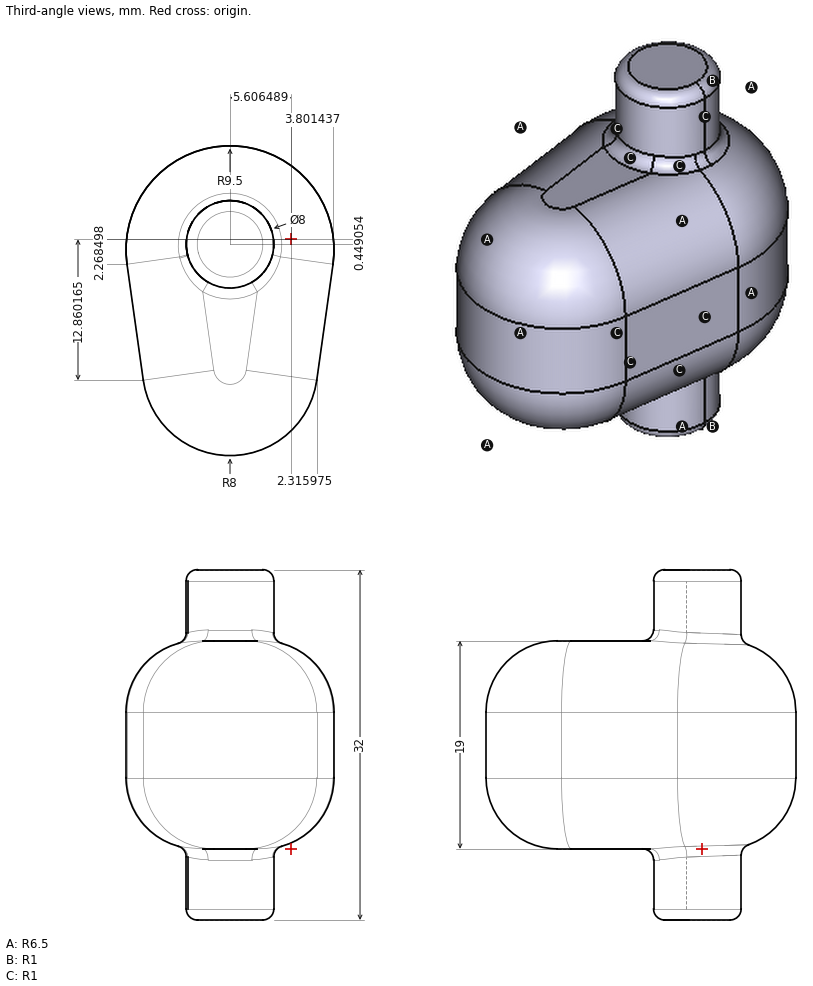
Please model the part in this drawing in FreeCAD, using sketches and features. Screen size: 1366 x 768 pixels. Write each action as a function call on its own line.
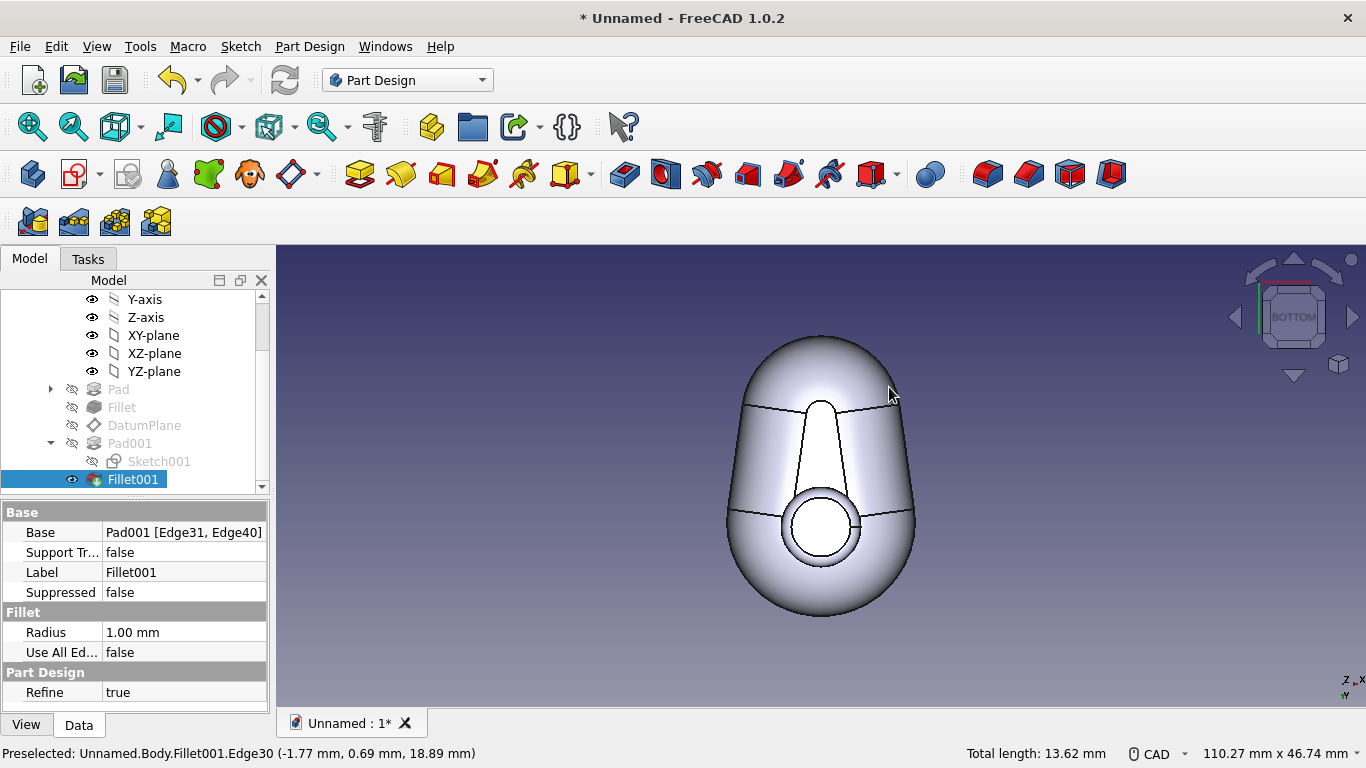
key(4)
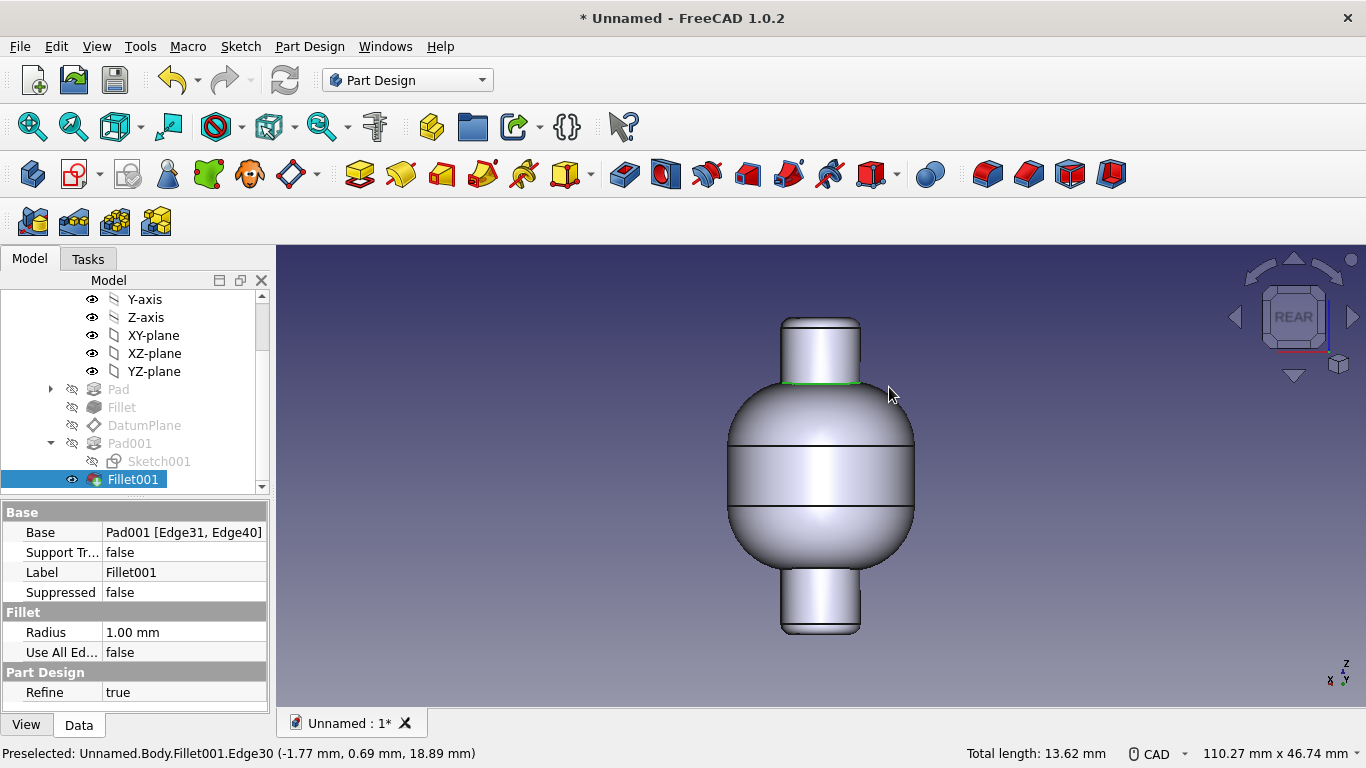
key(6)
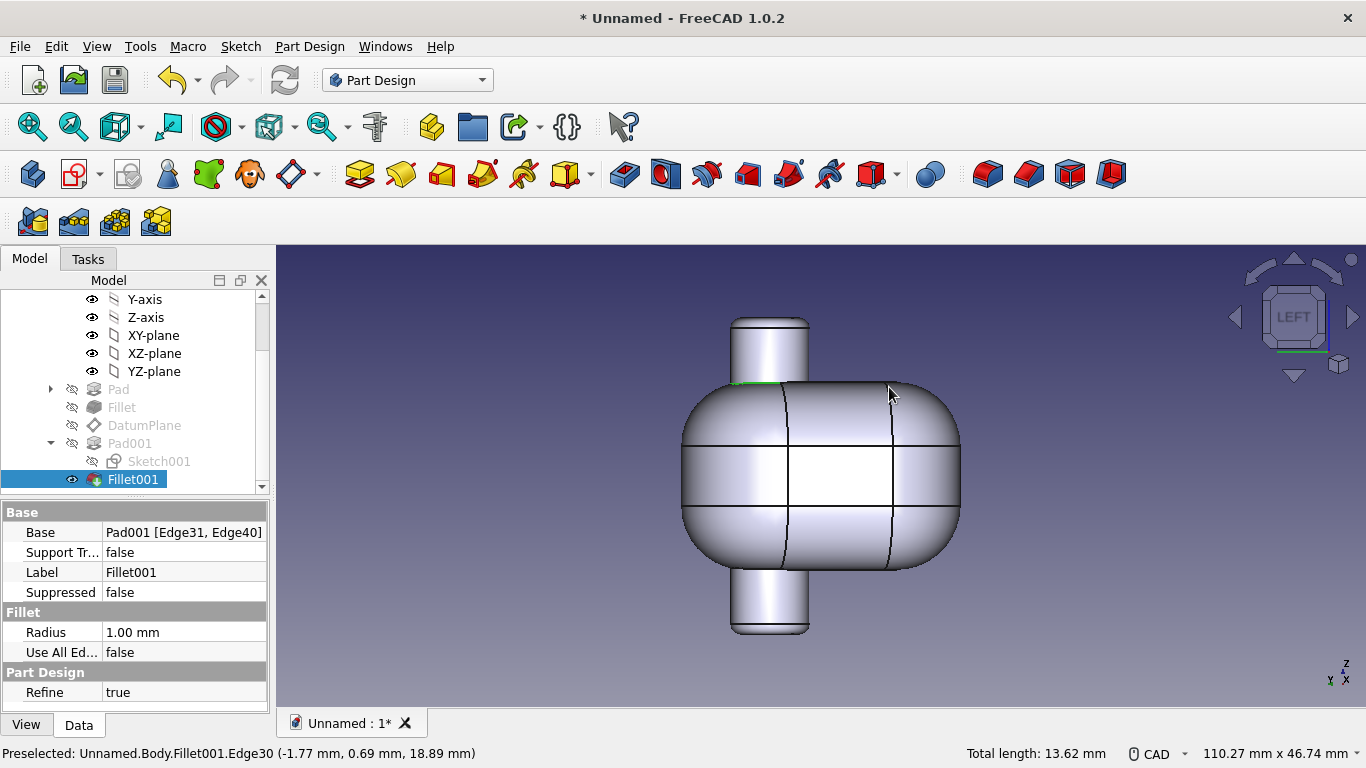
key(v)
key(3)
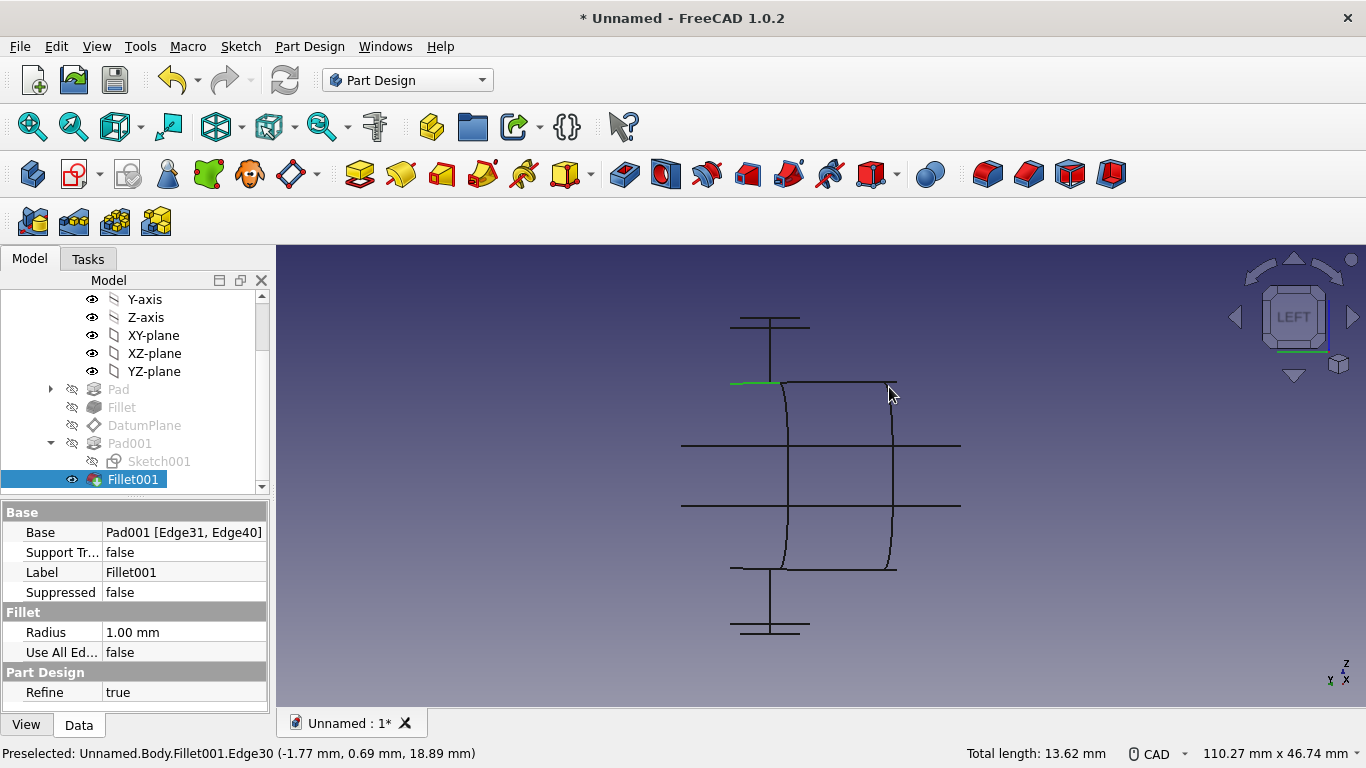
key(0)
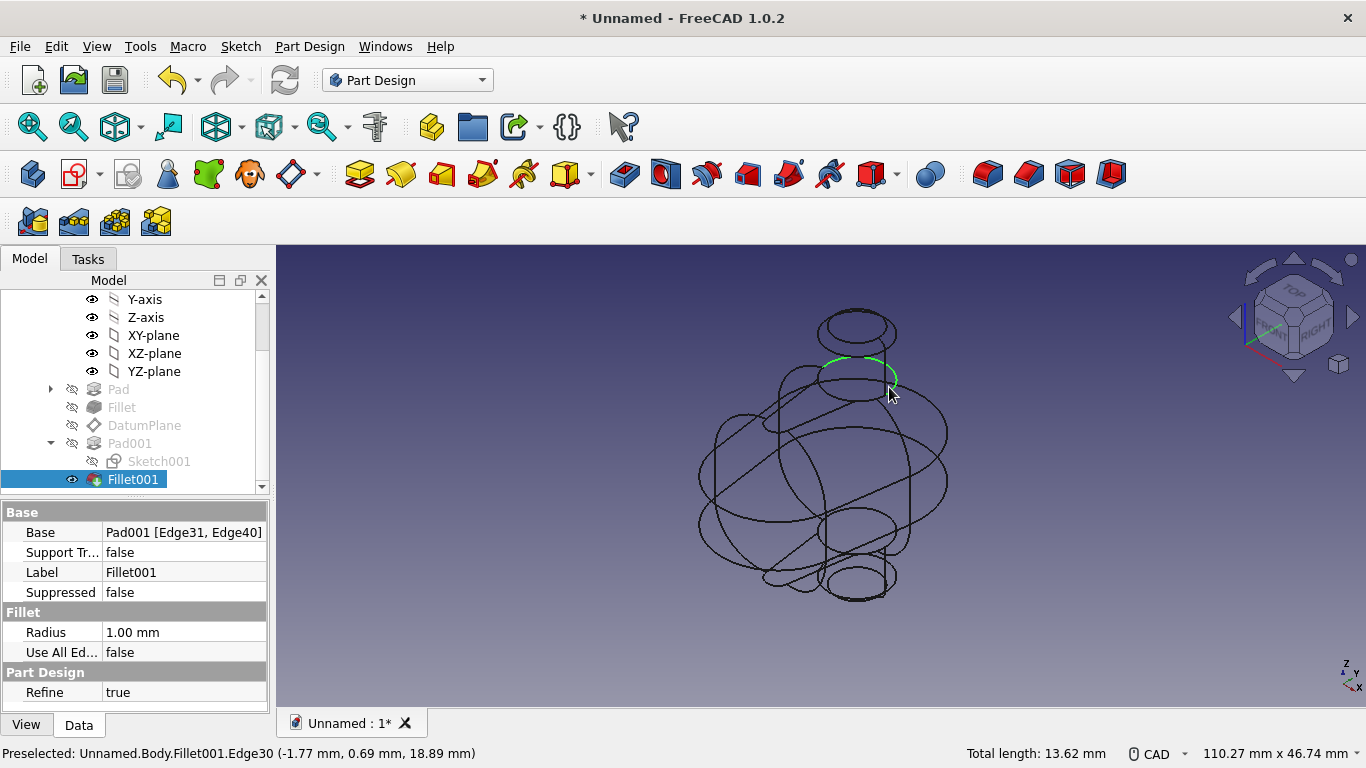
click(867, 400, ctrl)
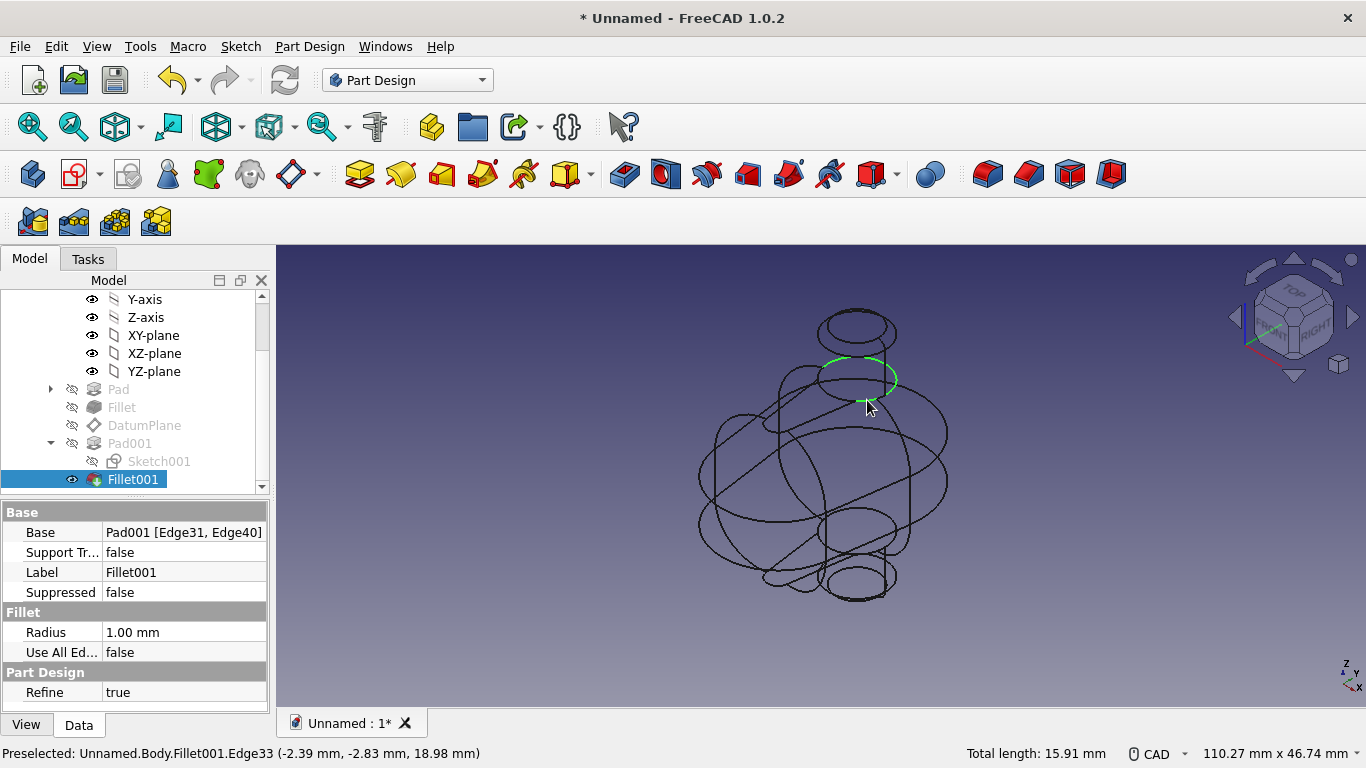
click(834, 549, ctrl)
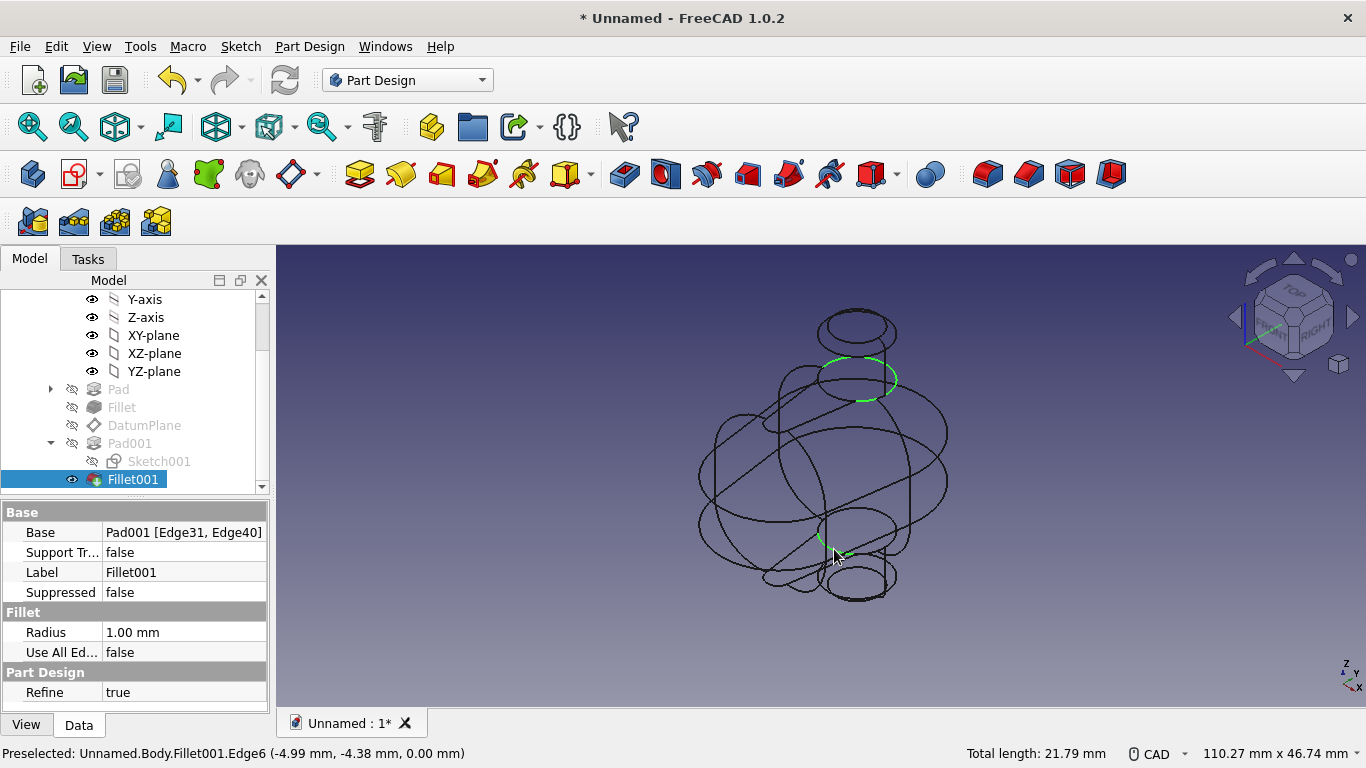
click(867, 553, ctrl)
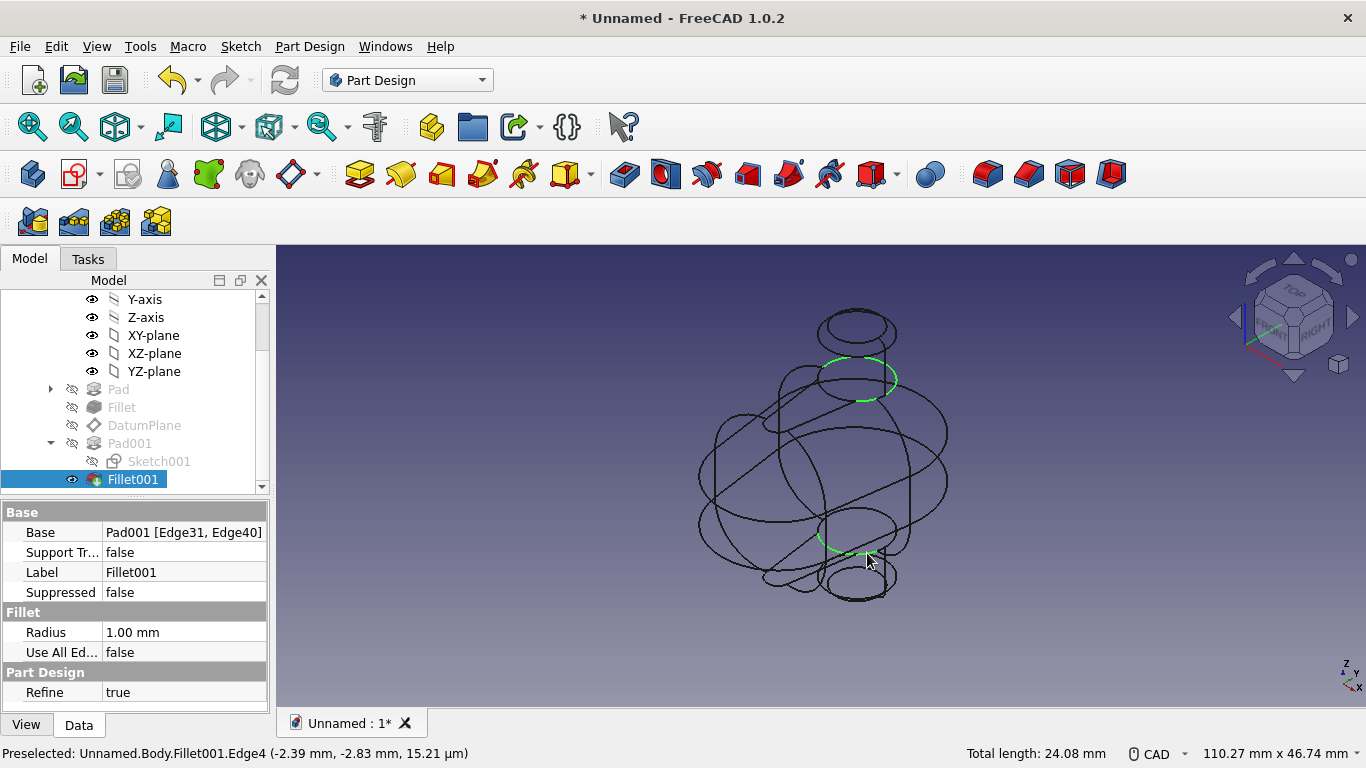
click(881, 511, ctrl)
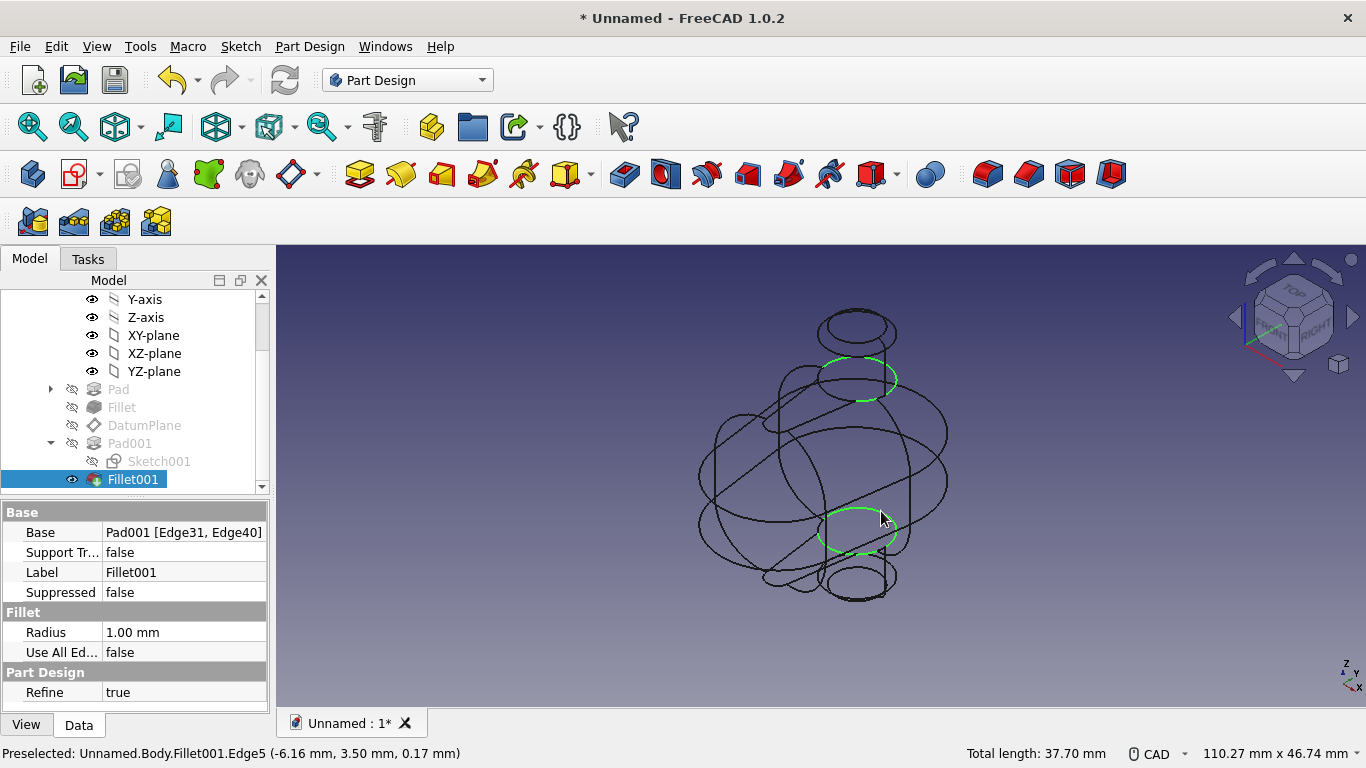
click(819, 525, ctrl)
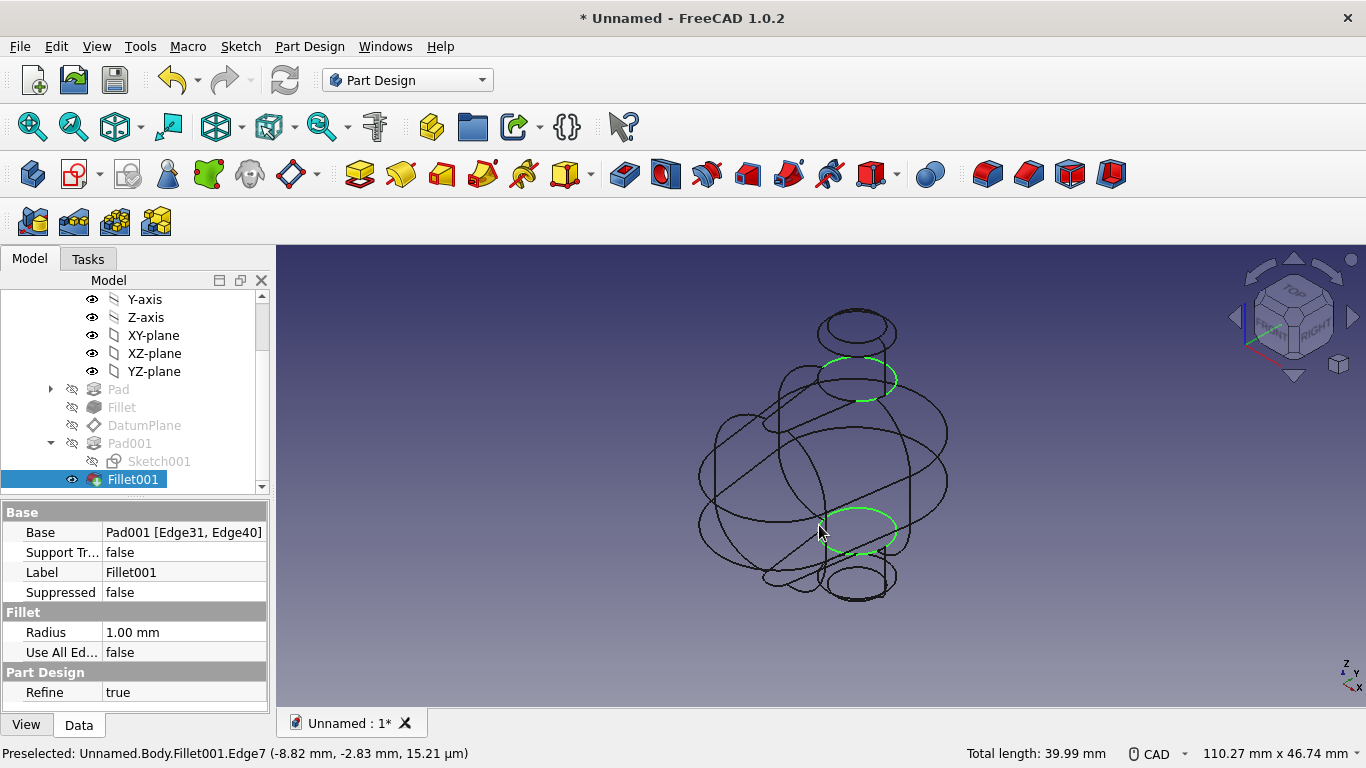
click(829, 394, ctrl)